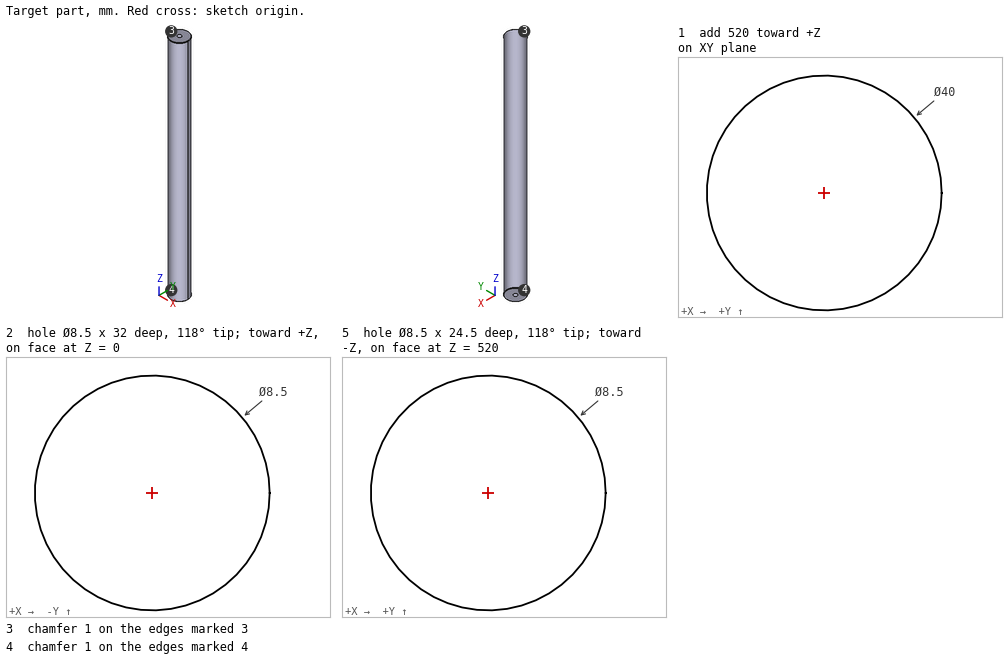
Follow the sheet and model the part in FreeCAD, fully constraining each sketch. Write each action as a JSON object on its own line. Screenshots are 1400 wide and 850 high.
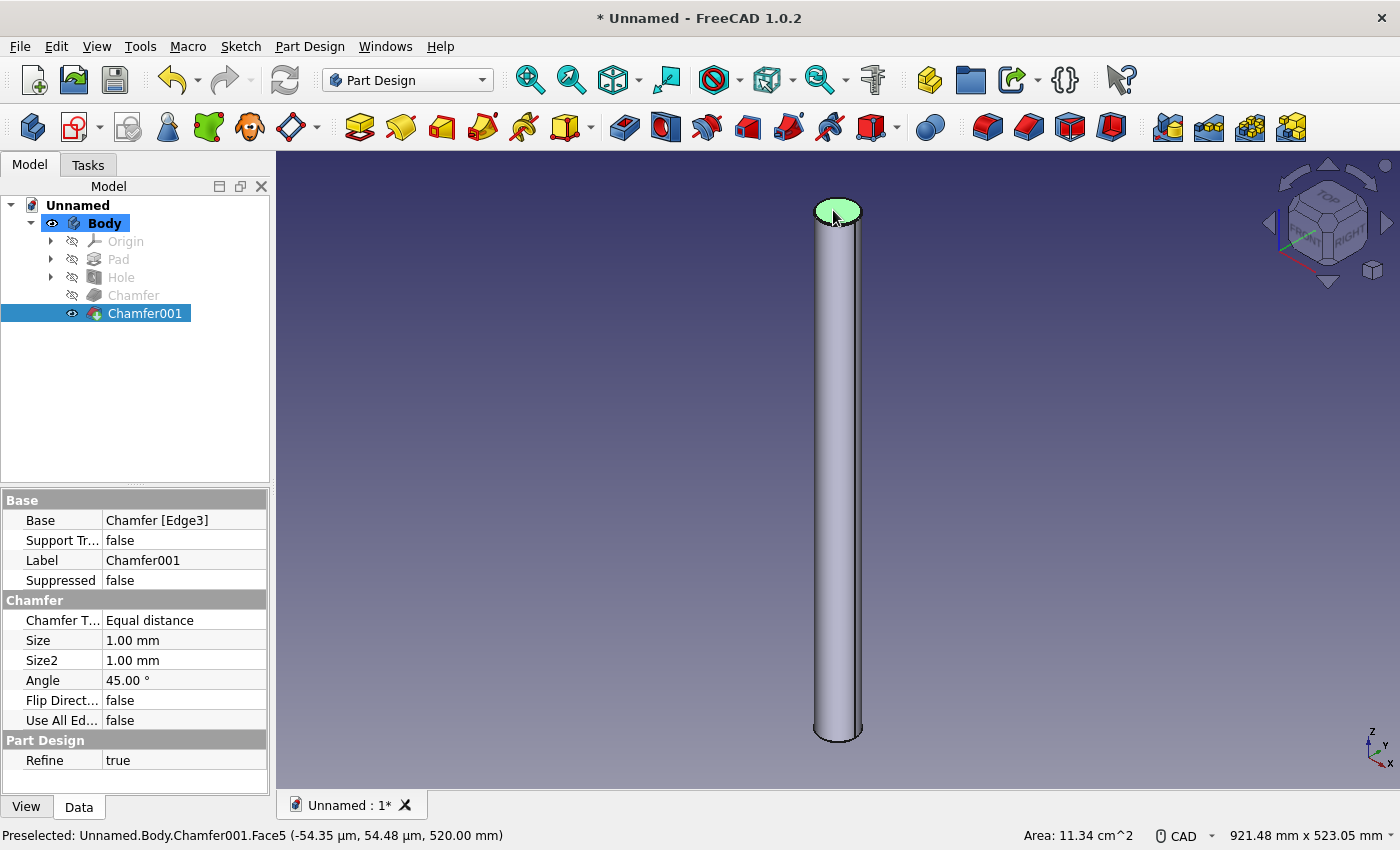
{"action": "left_click", "coordinate": [74, 128]}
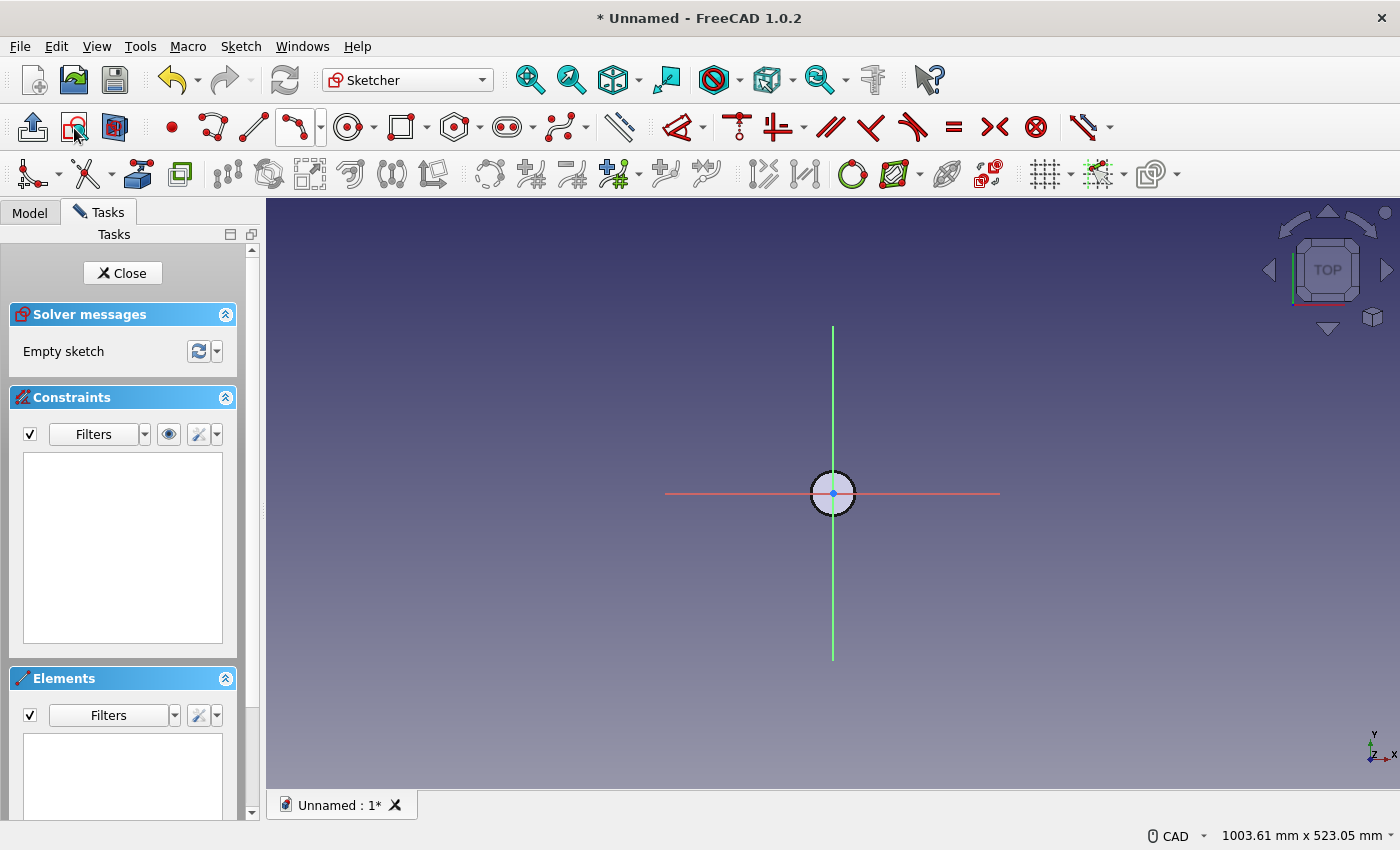
{"action": "scroll", "coordinate": [837, 494], "scroll_direction": "up", "scroll_amount": 15}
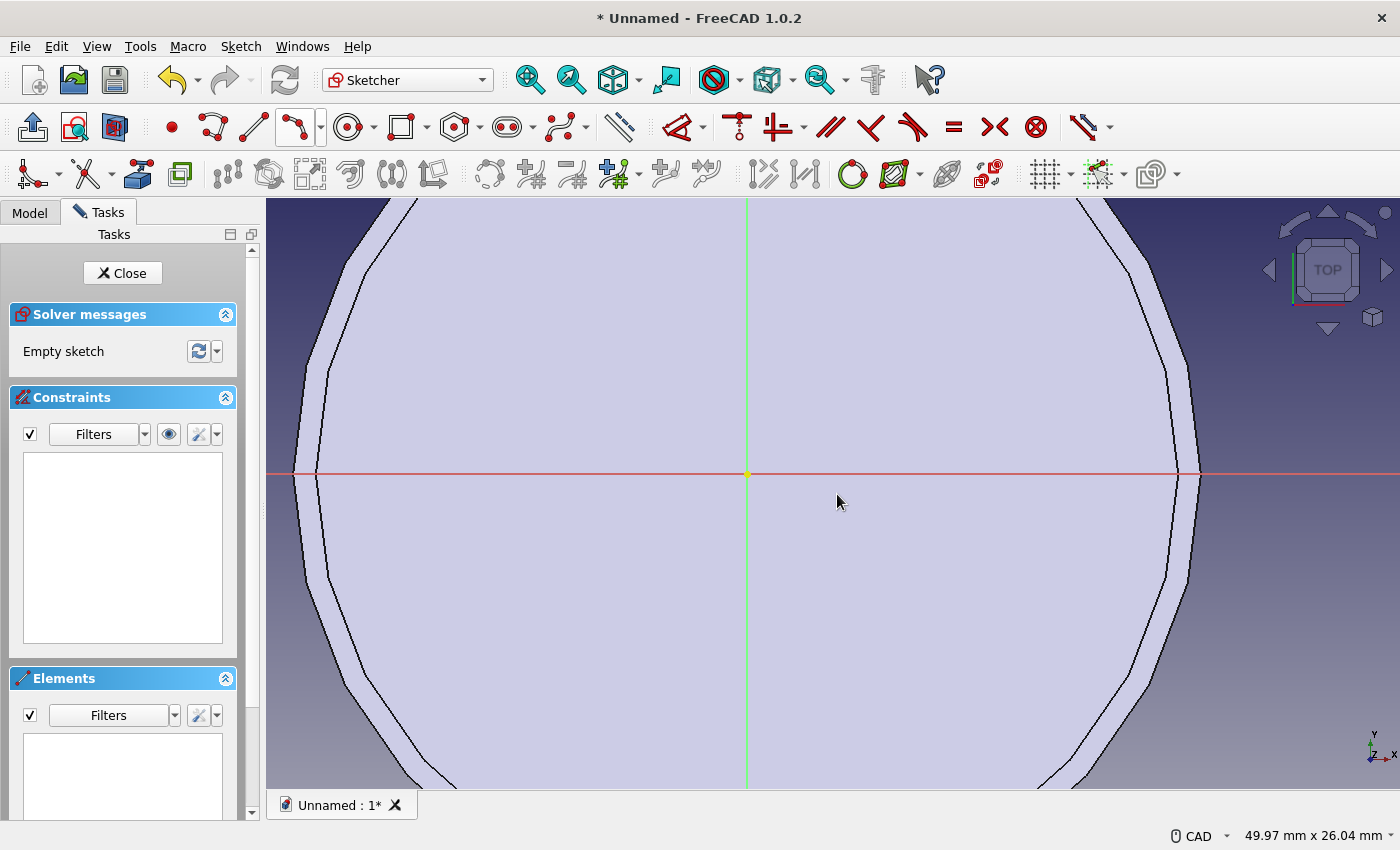
{"action": "scroll", "coordinate": [726, 451], "scroll_direction": "up", "scroll_amount": 3}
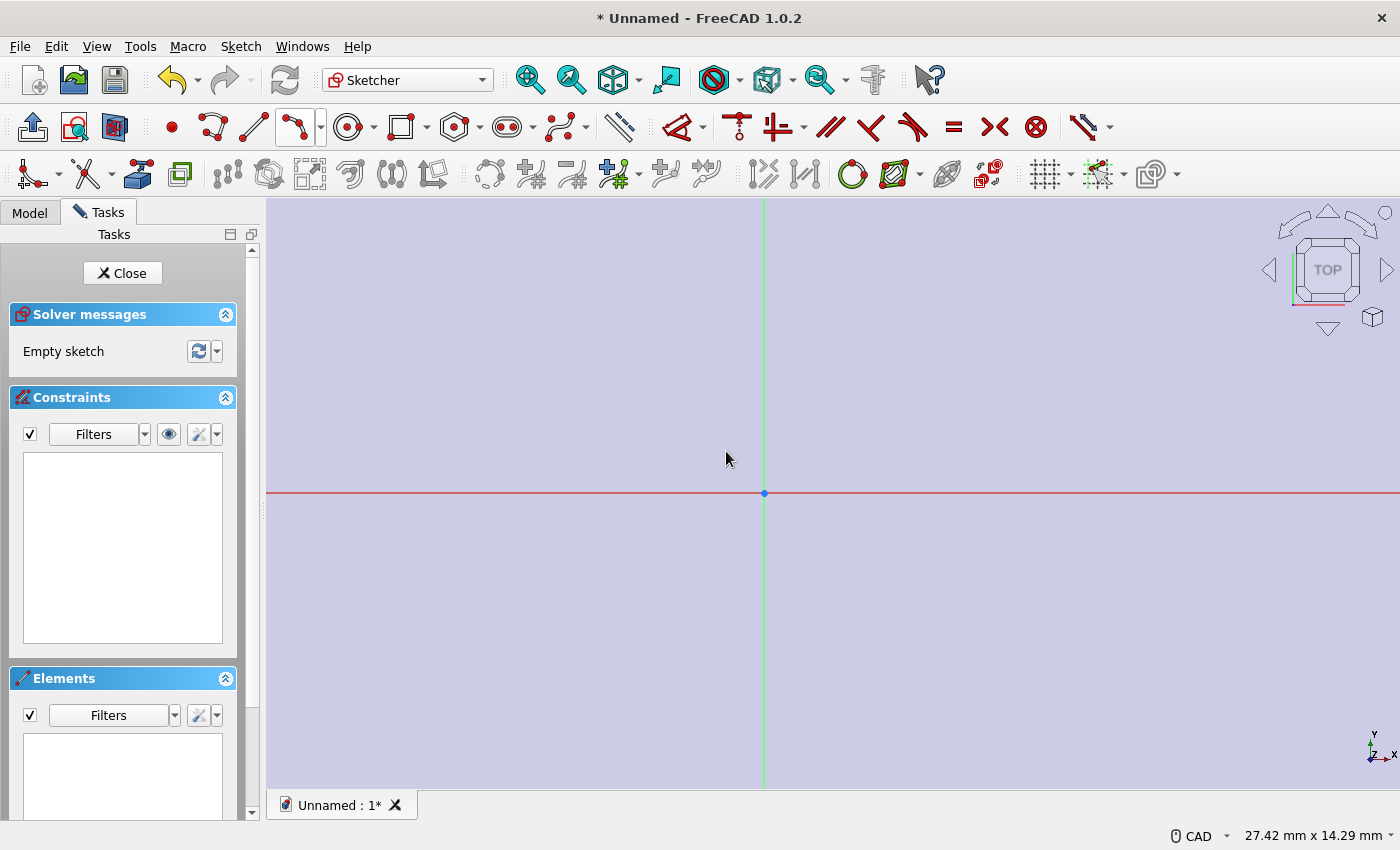
{"action": "left_click", "coordinate": [348, 128]}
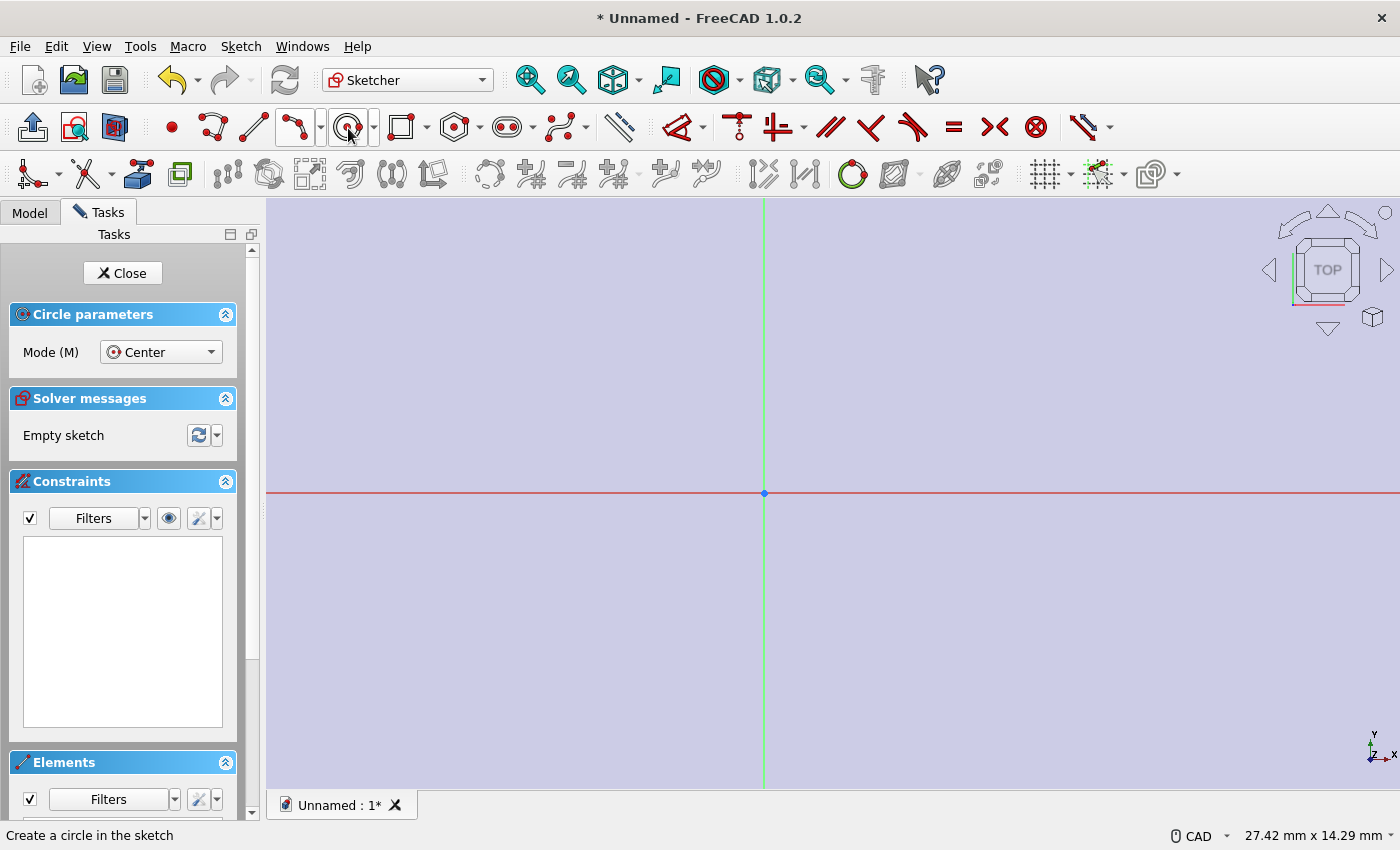
{"action": "left_click", "coordinate": [764, 493]}
{"action": "left_click", "coordinate": [888, 369]}
{"action": "key", "text": "Escape"}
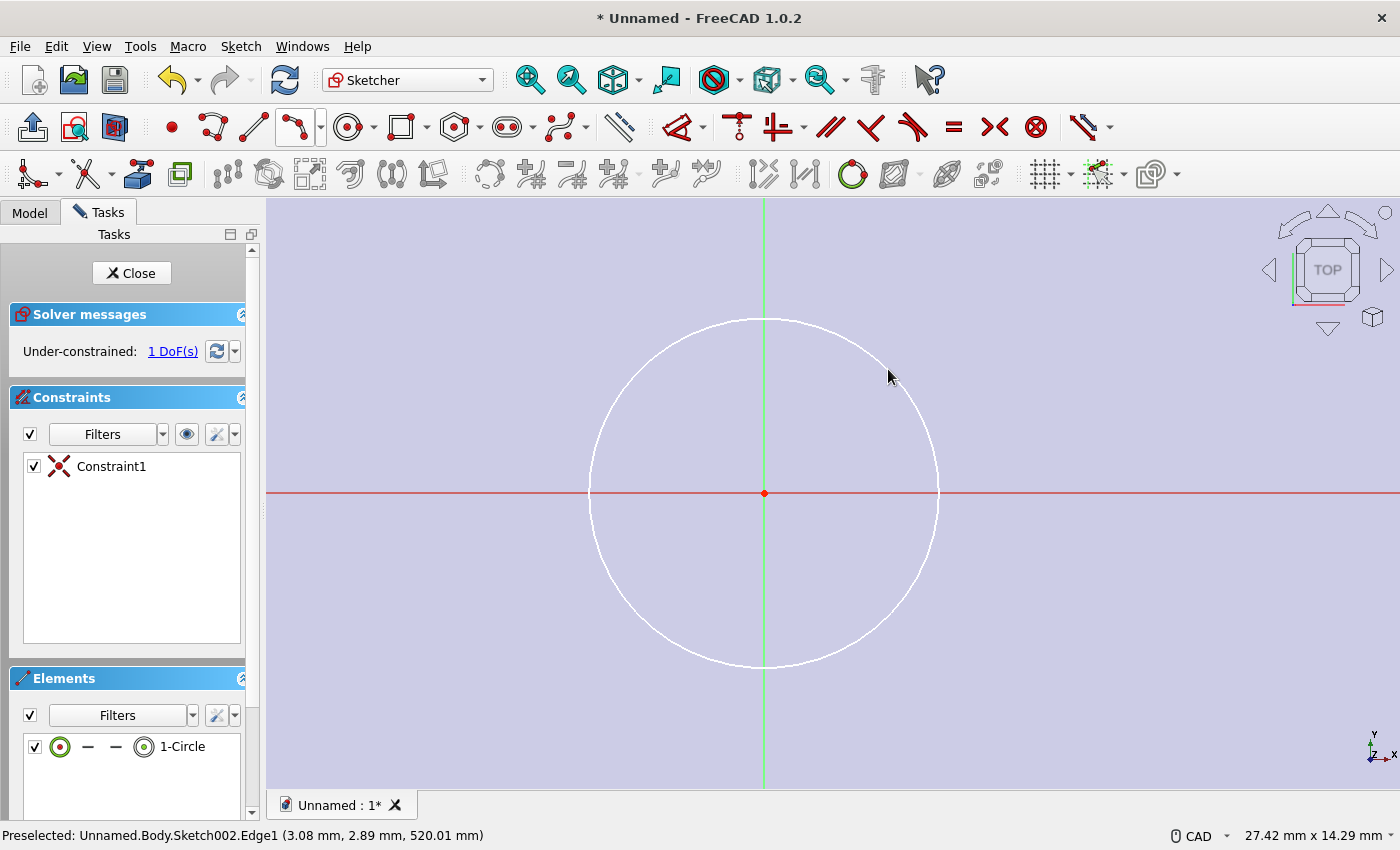
{"action": "left_click", "coordinate": [676, 128]}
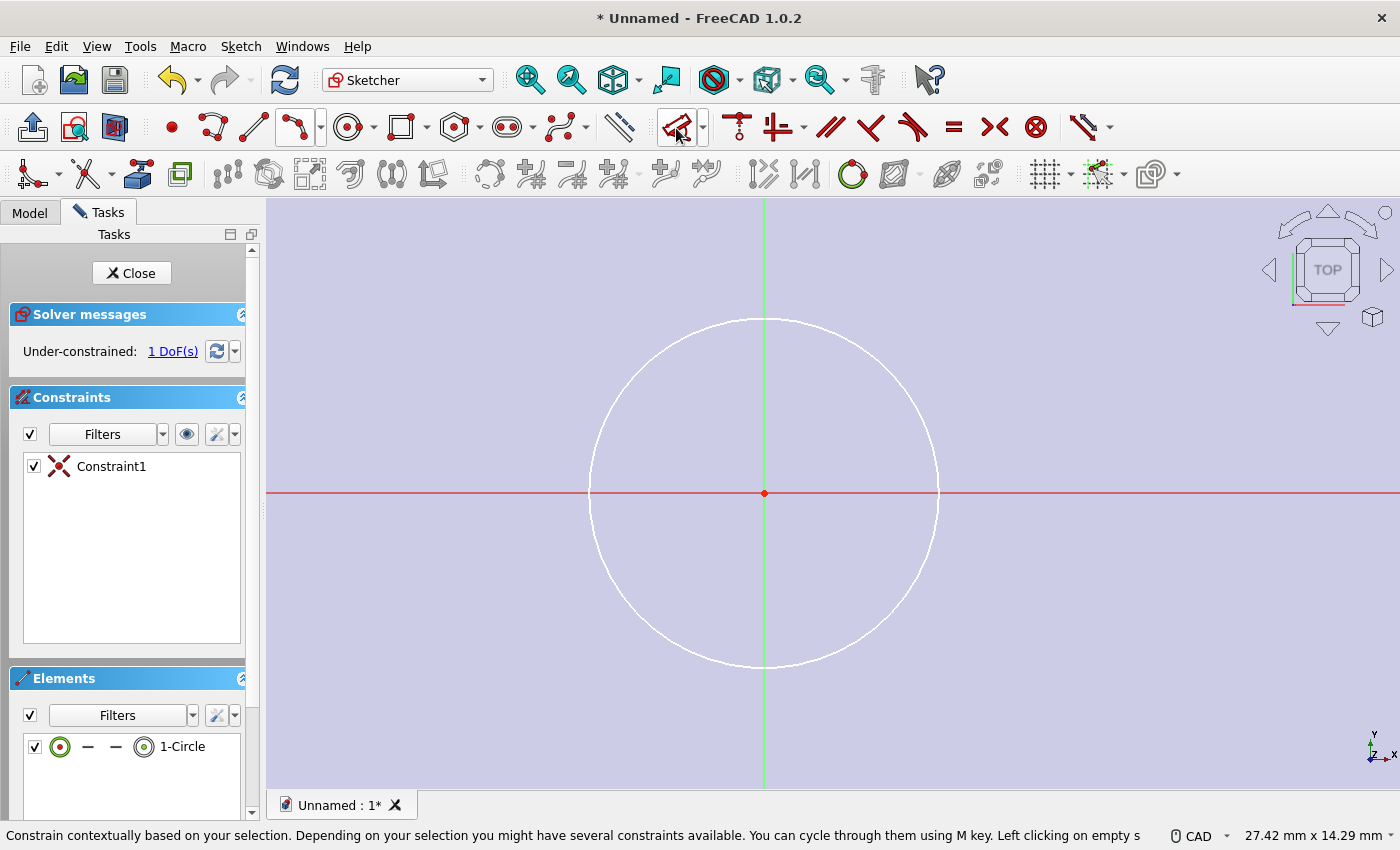
{"action": "left_click", "coordinate": [887, 369]}
{"action": "left_click", "coordinate": [910, 346]}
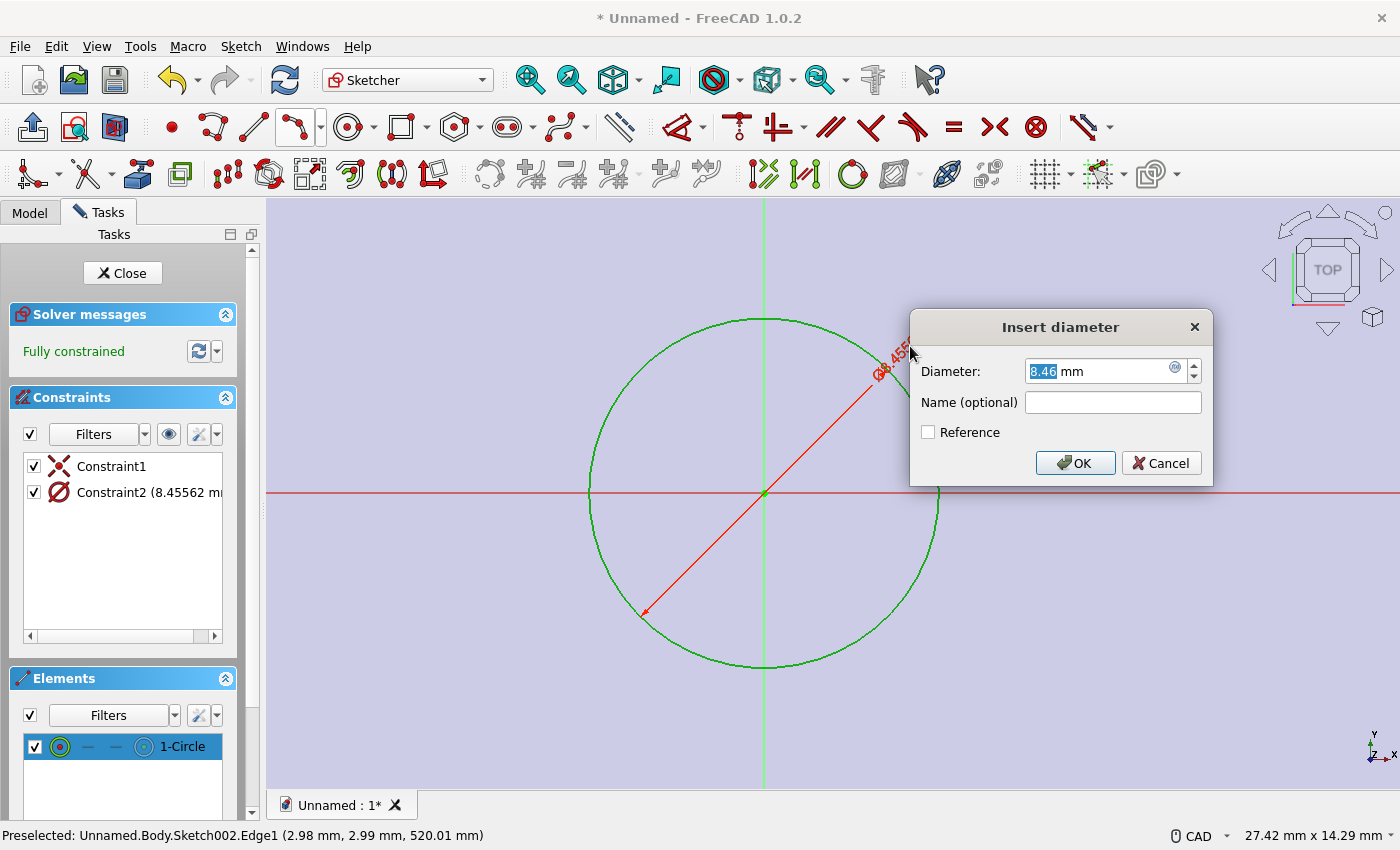
{"action": "type", "text": "8.5"}
{"action": "key", "text": "Return"}
{"action": "key", "text": "Escape"}